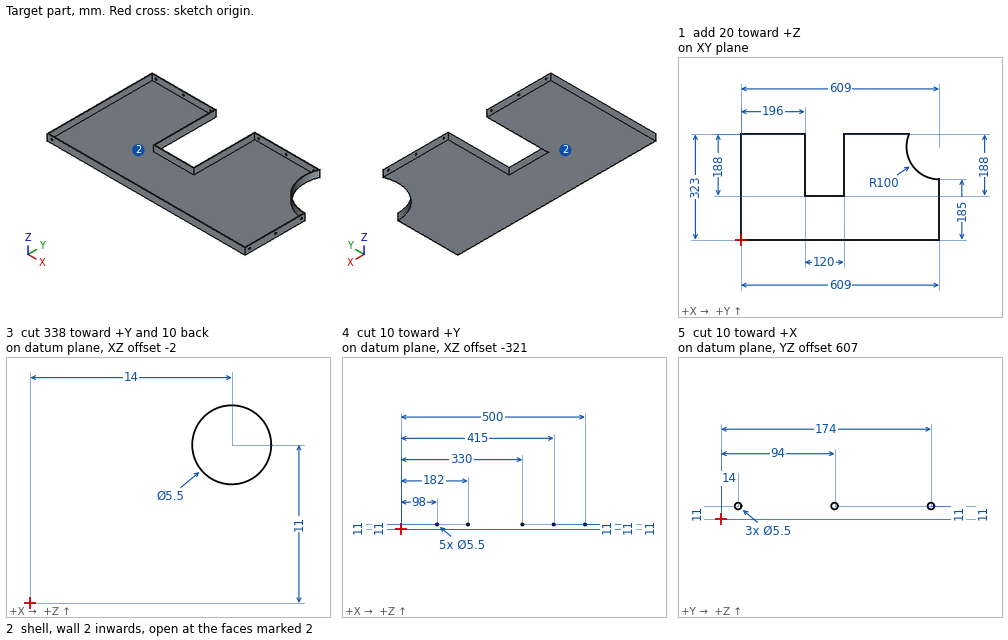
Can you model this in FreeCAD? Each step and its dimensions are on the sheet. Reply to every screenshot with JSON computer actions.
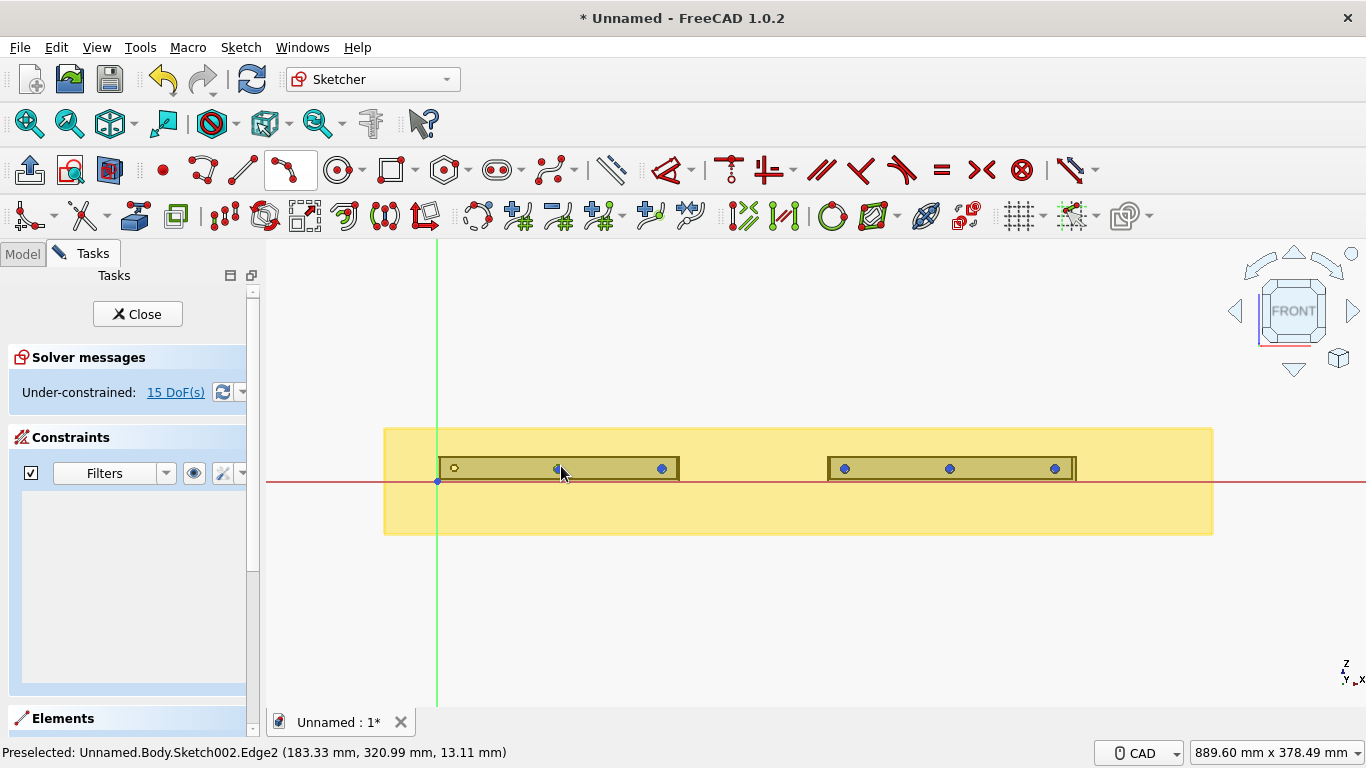
{"action": "scroll", "coordinate": [848, 466], "scroll_direction": "up", "scroll_amount": 7}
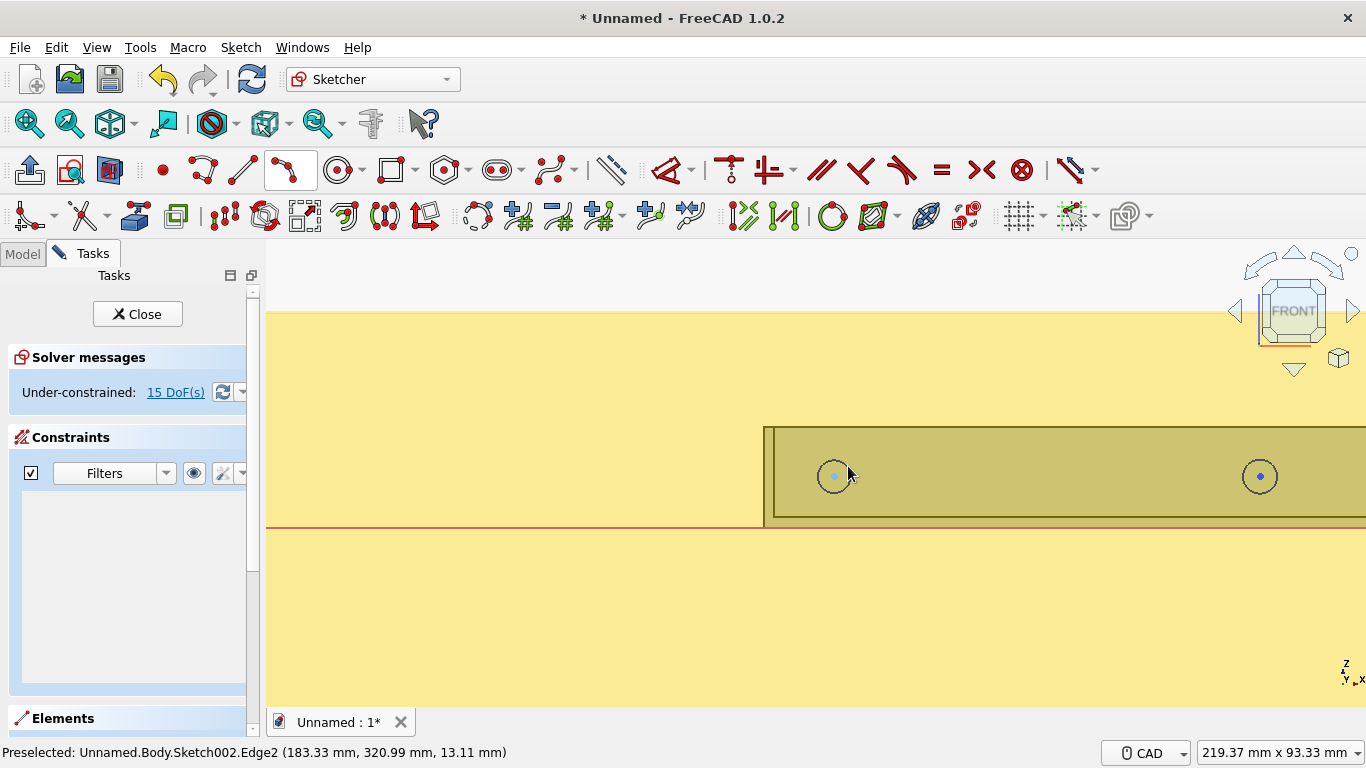
{"action": "left_click", "coordinate": [846, 465]}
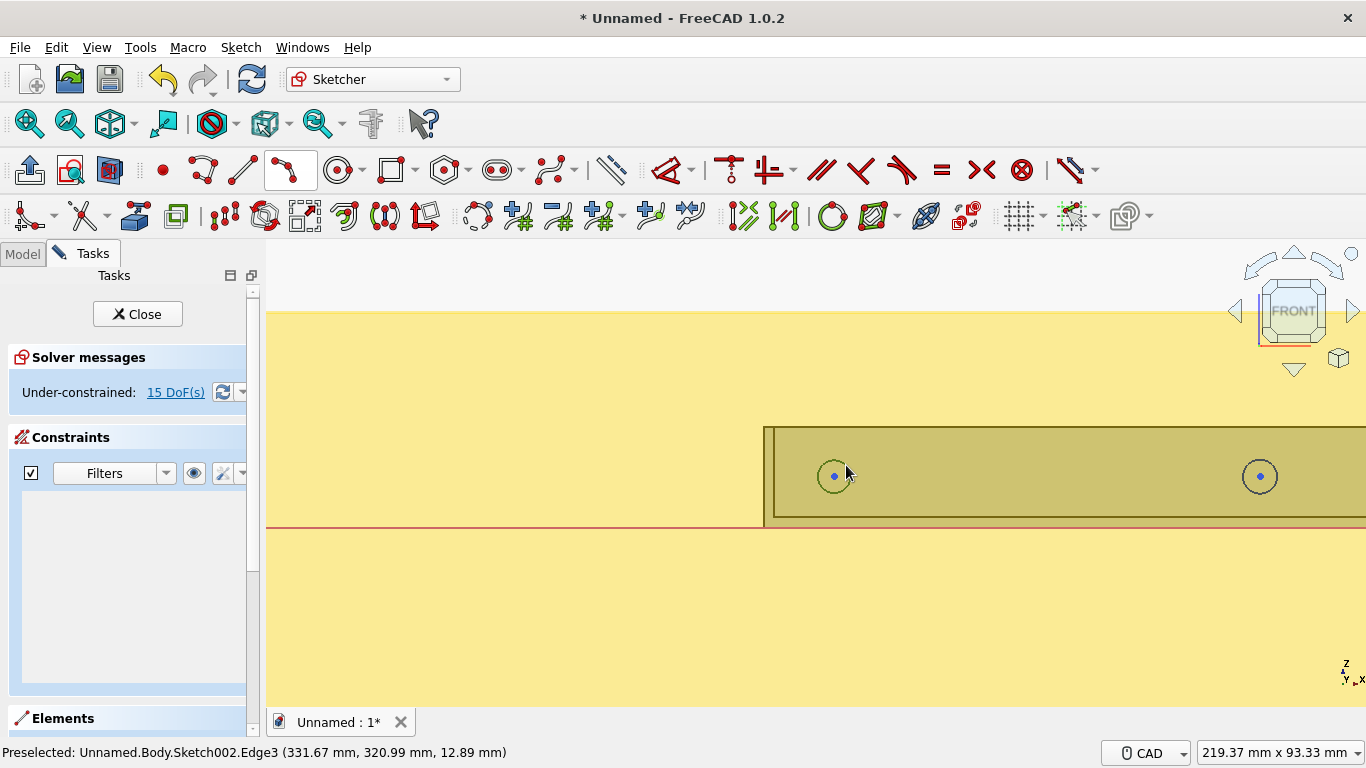
{"action": "scroll", "coordinate": [848, 466], "scroll_direction": "down", "scroll_amount": 7}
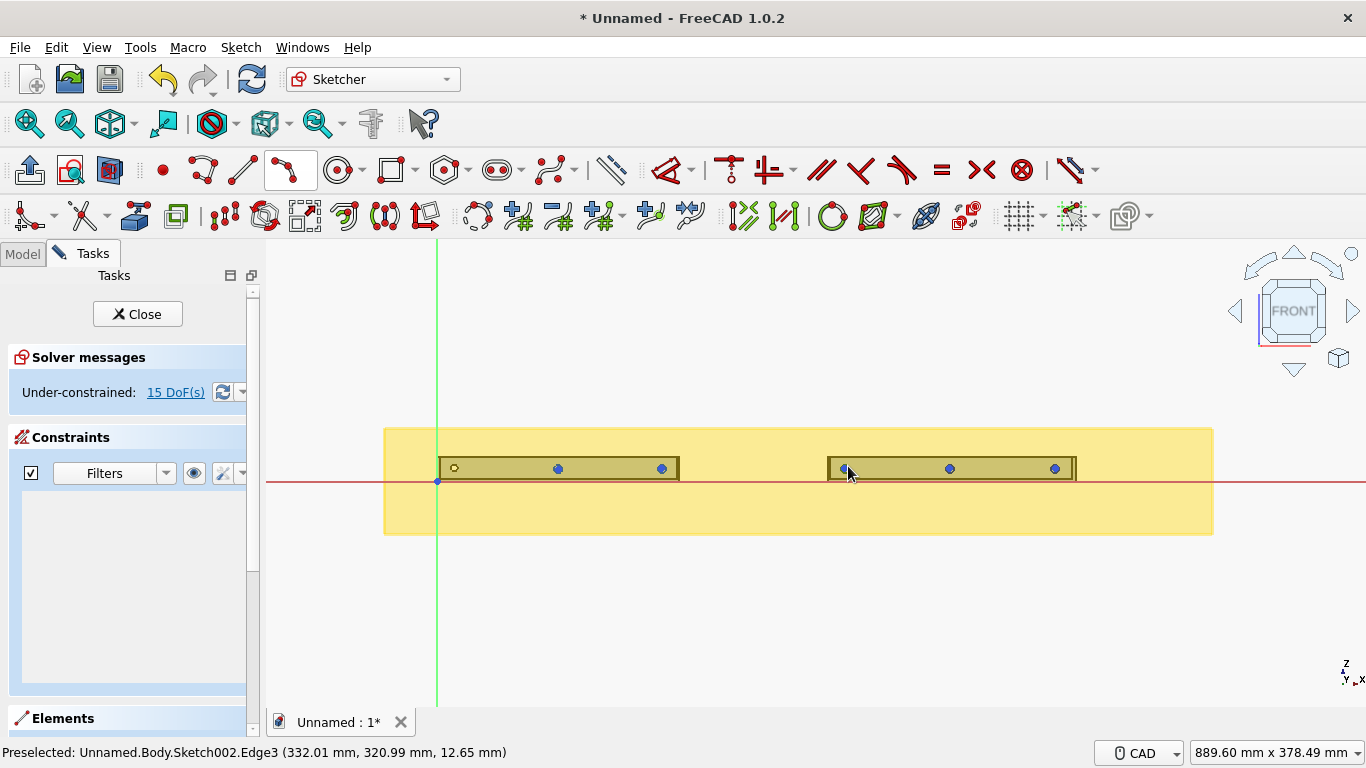
{"action": "scroll", "coordinate": [953, 466], "scroll_direction": "up", "scroll_amount": 6}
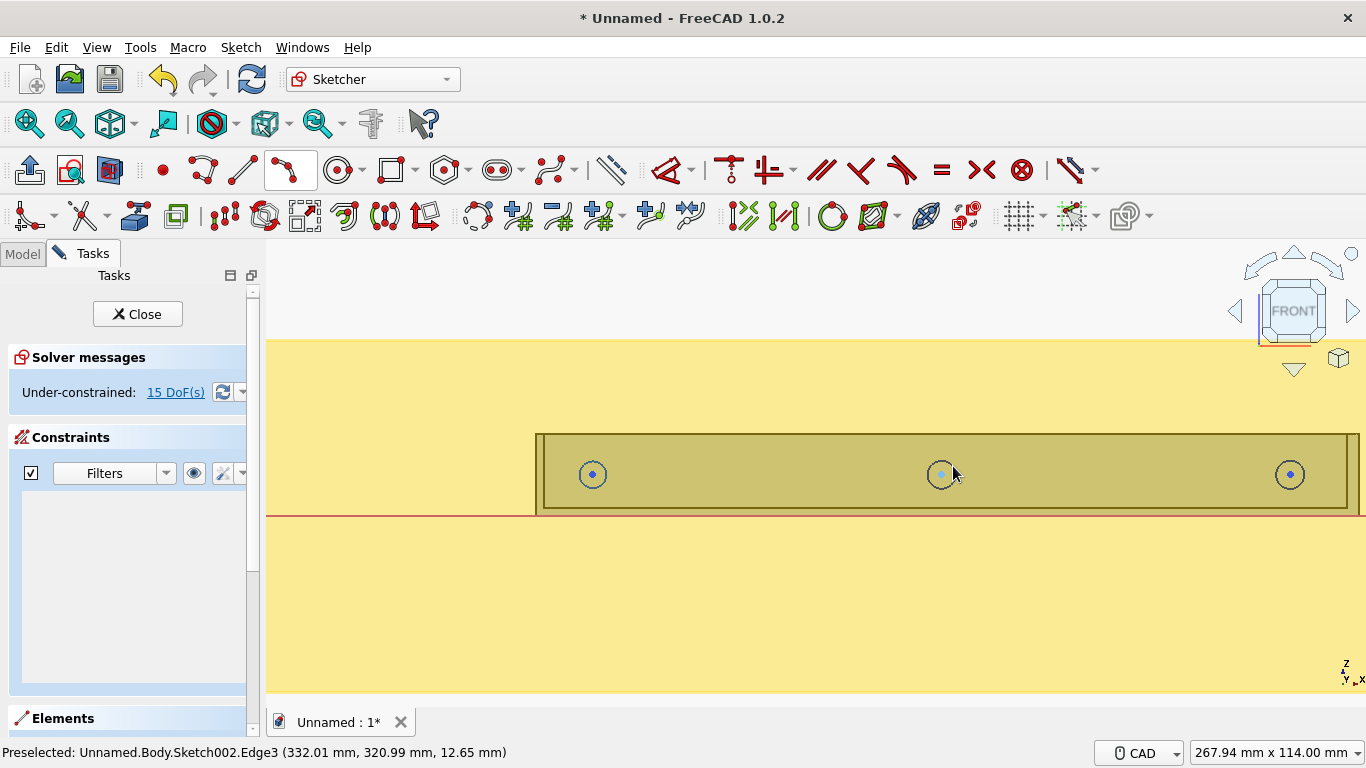
{"action": "left_click", "coordinate": [951, 465]}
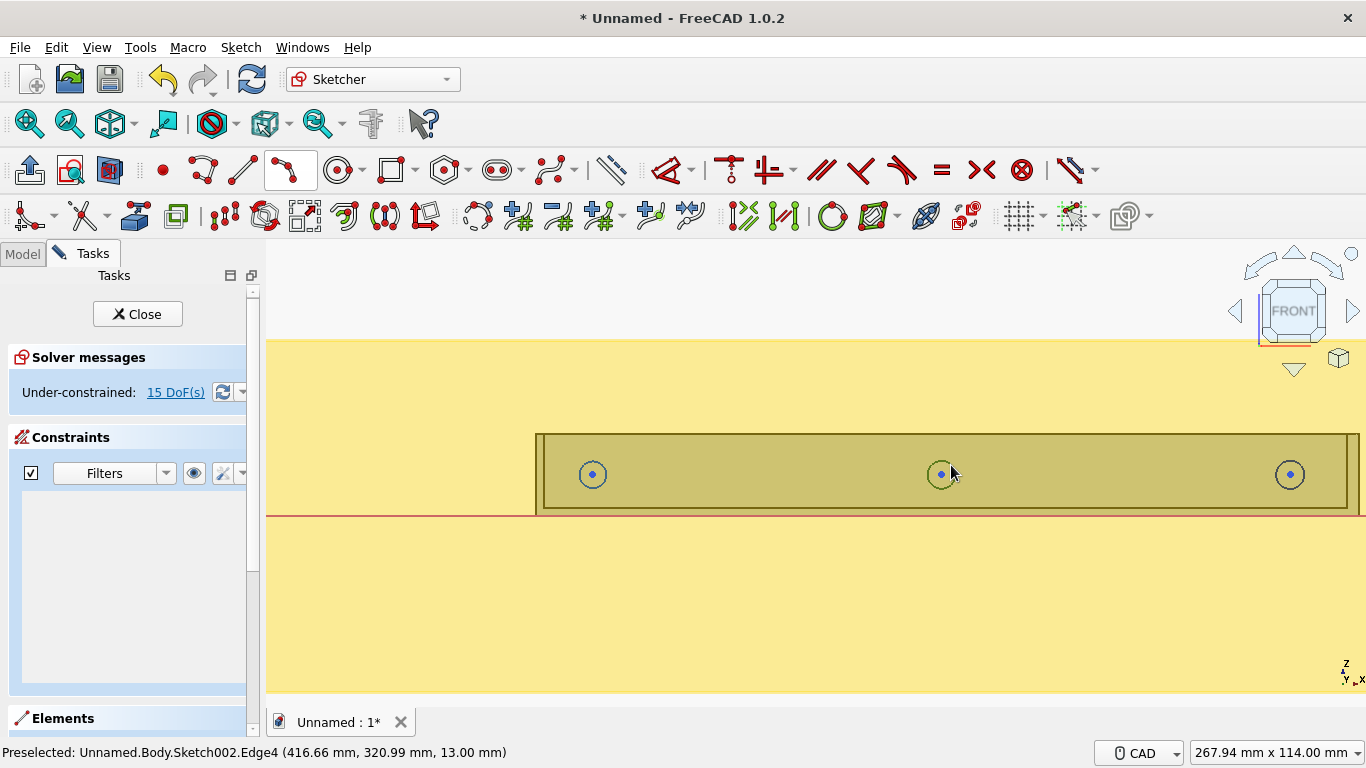
{"action": "scroll", "coordinate": [953, 466], "scroll_direction": "down", "scroll_amount": 6}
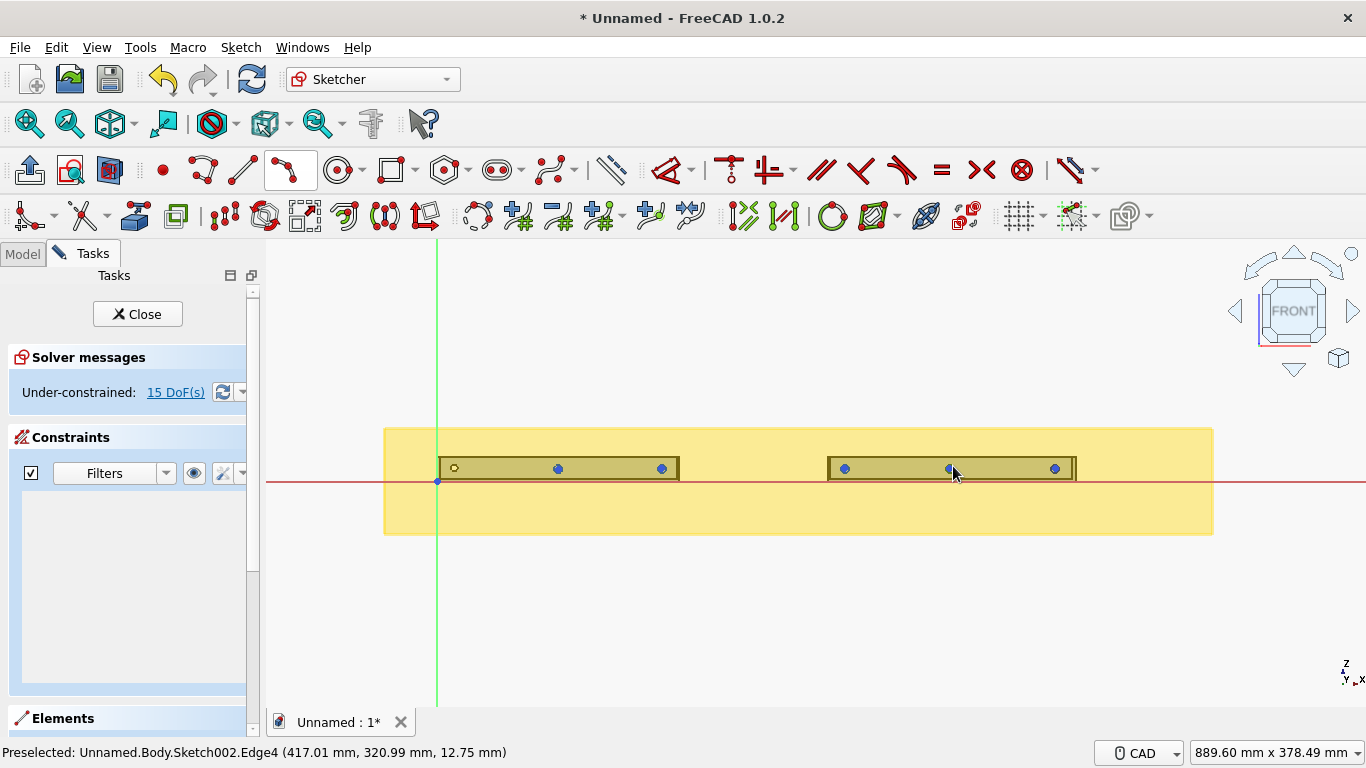
{"action": "scroll", "coordinate": [1058, 466], "scroll_direction": "up", "scroll_amount": 6}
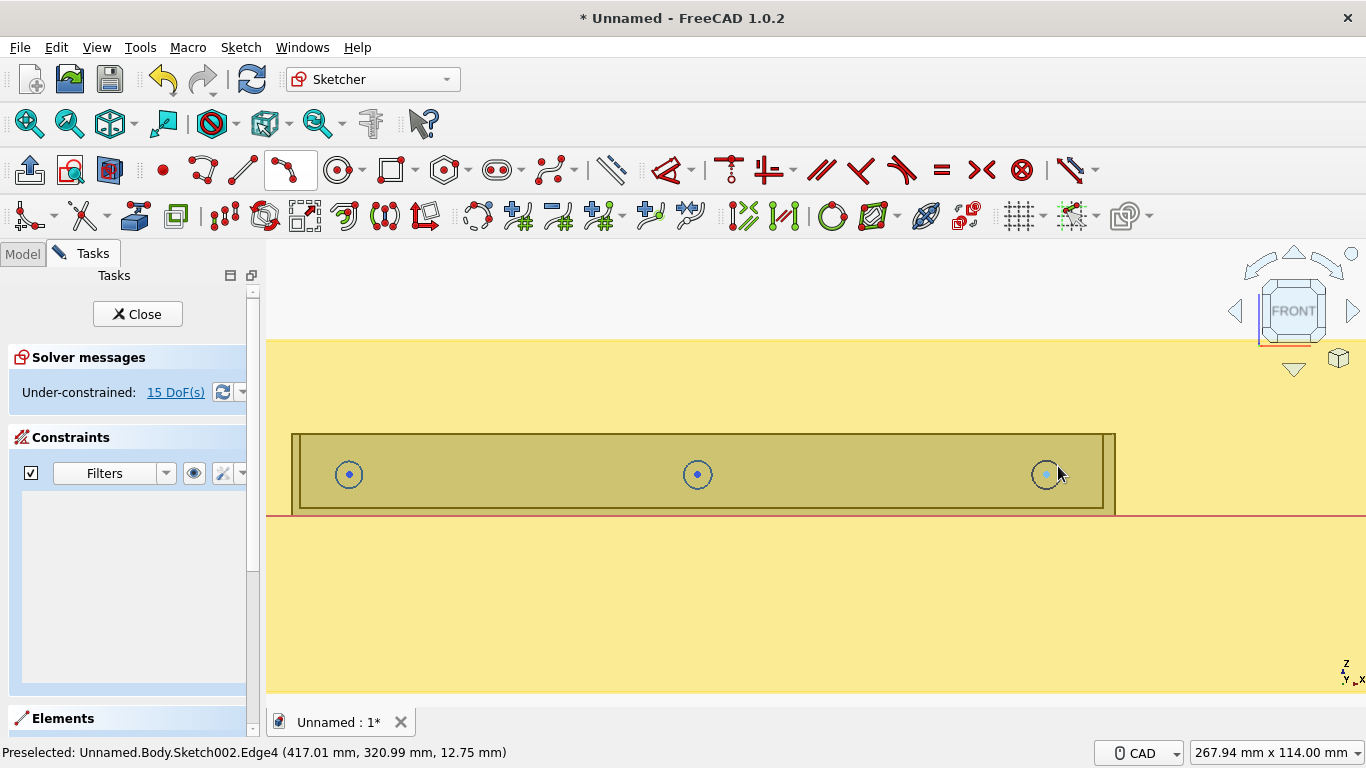
{"action": "left_click", "coordinate": [1056, 465]}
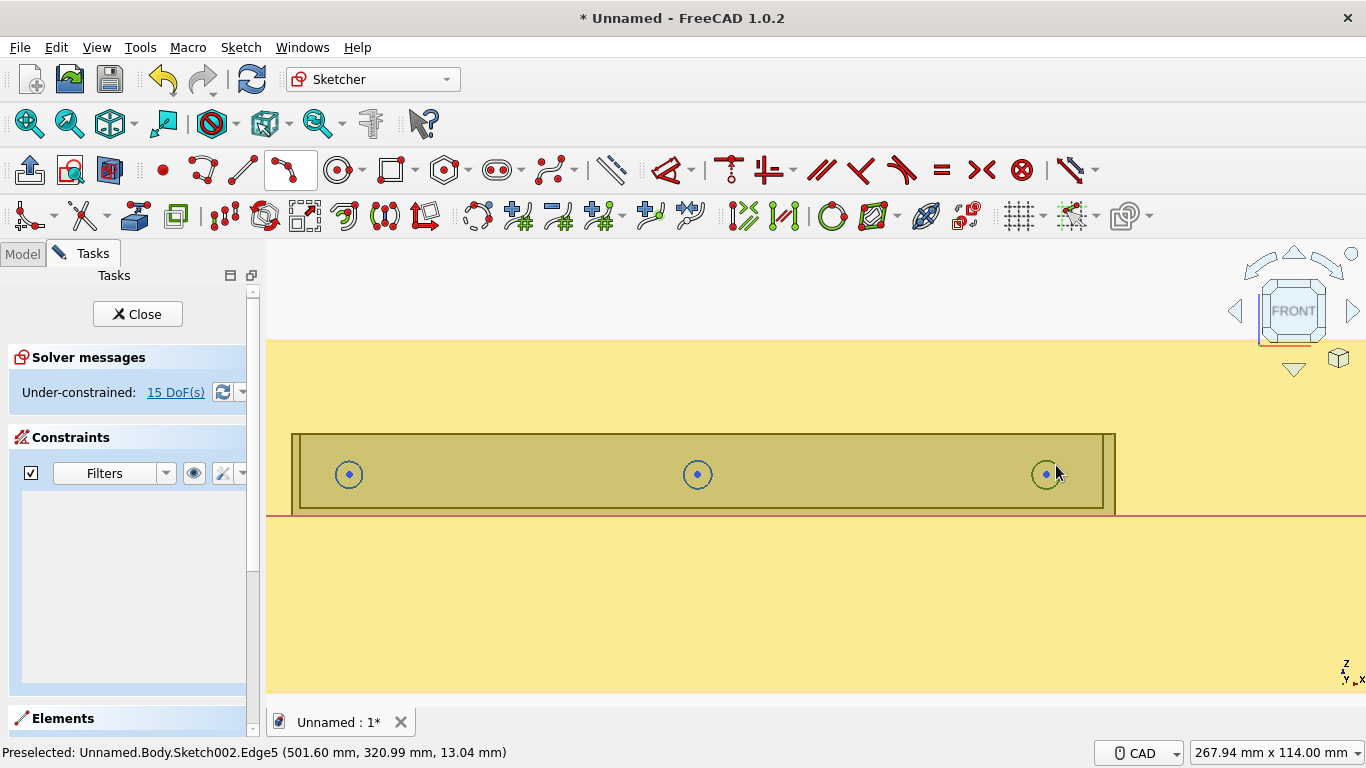
{"action": "key", "text": "e"}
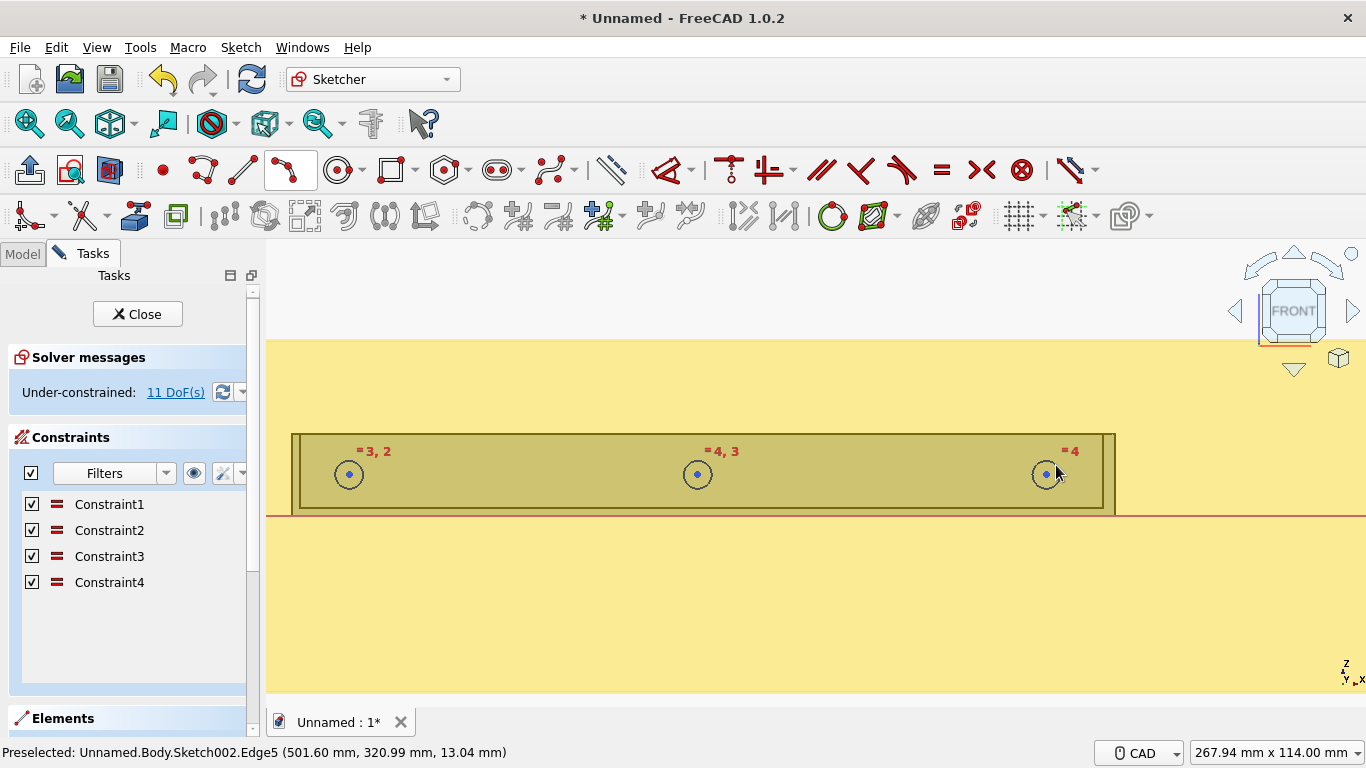
{"action": "scroll", "coordinate": [1058, 466], "scroll_direction": "down", "scroll_amount": 6}